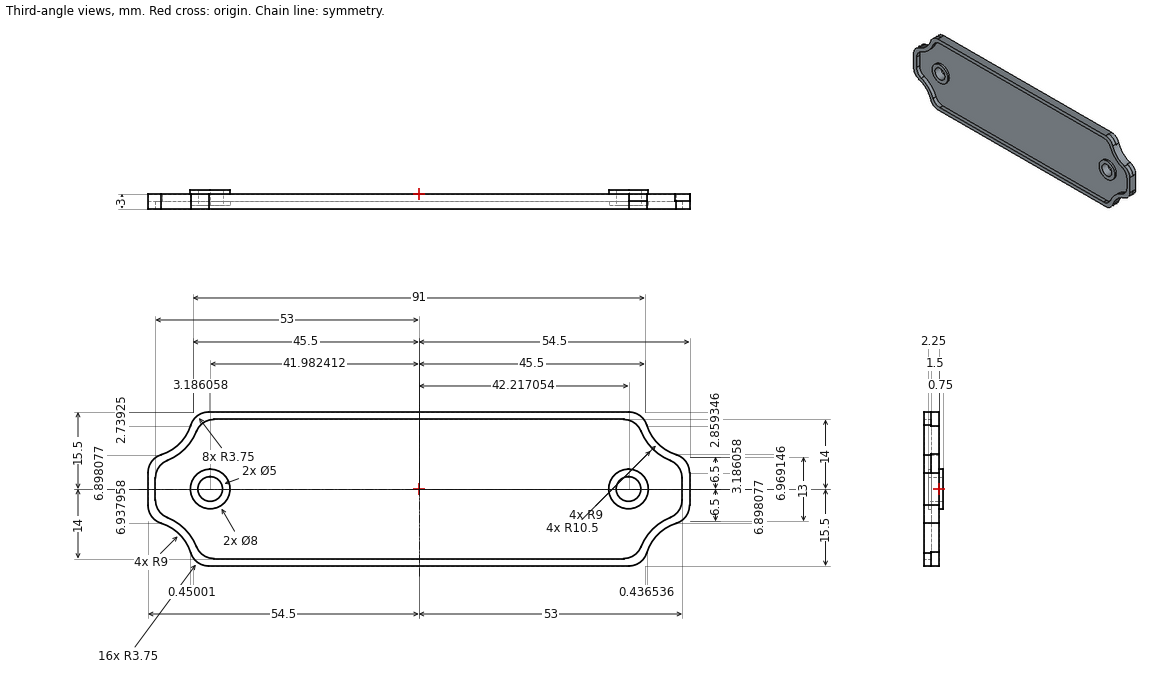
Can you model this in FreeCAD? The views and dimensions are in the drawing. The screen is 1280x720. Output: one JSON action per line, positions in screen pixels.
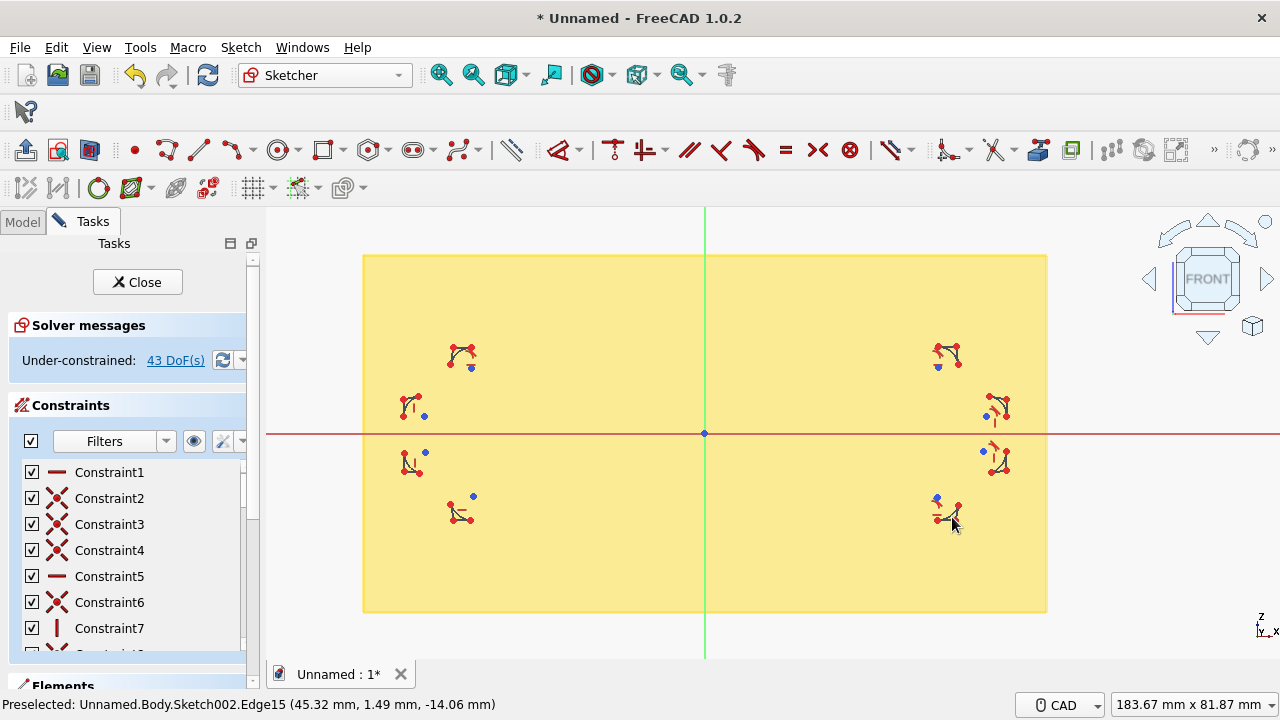
{"action": "scroll", "coordinate": [459, 520], "scroll_direction": "up", "scroll_amount": 7}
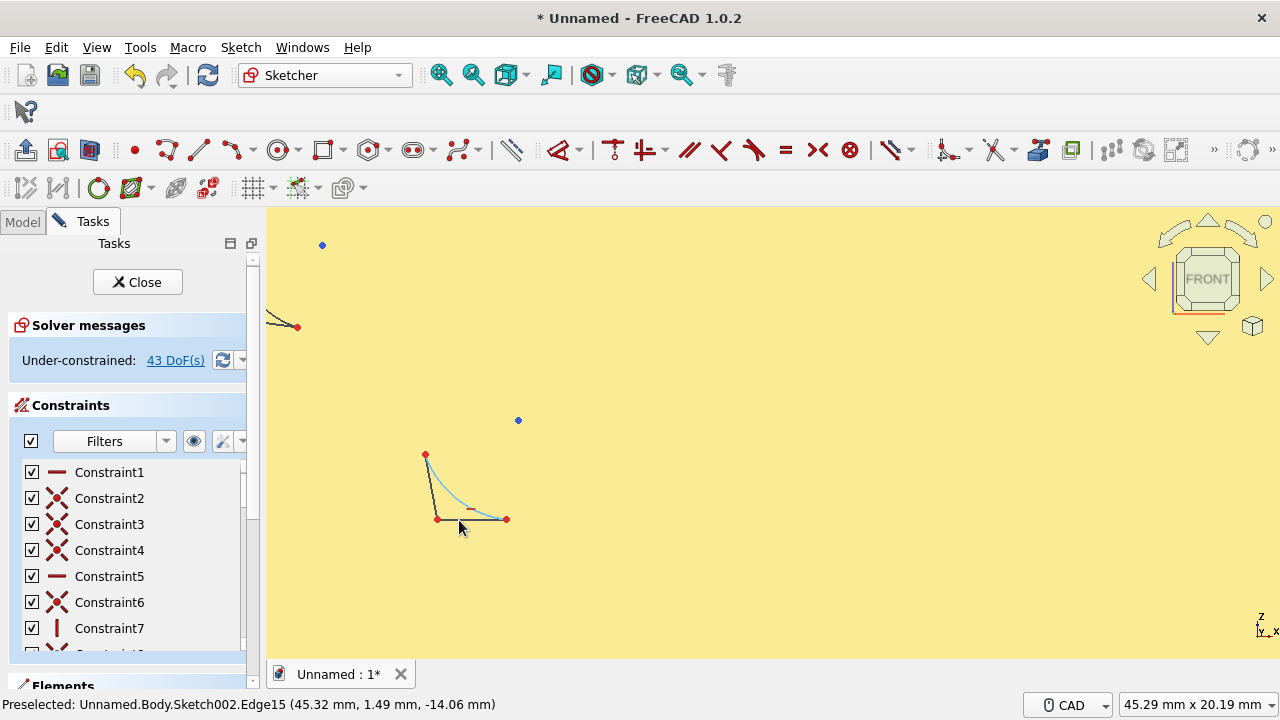
{"action": "left_click", "coordinate": [458, 520]}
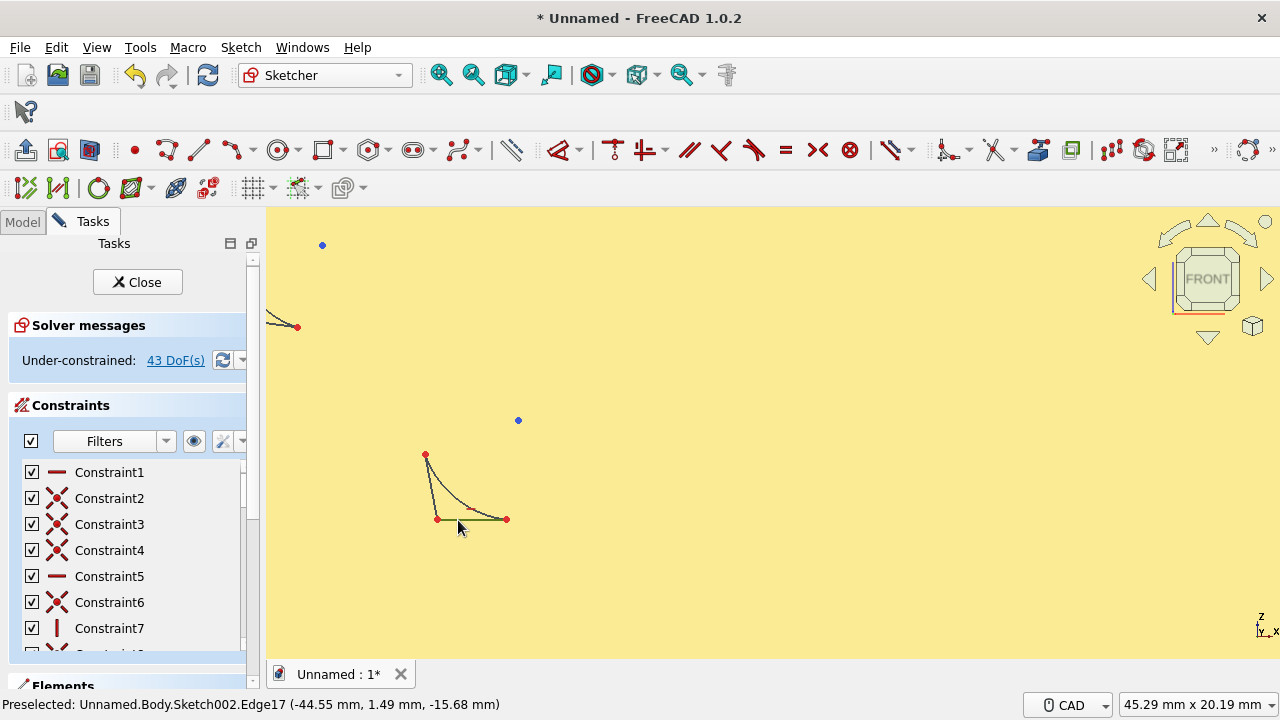
{"action": "scroll", "coordinate": [441, 483], "scroll_direction": "up", "scroll_amount": 2}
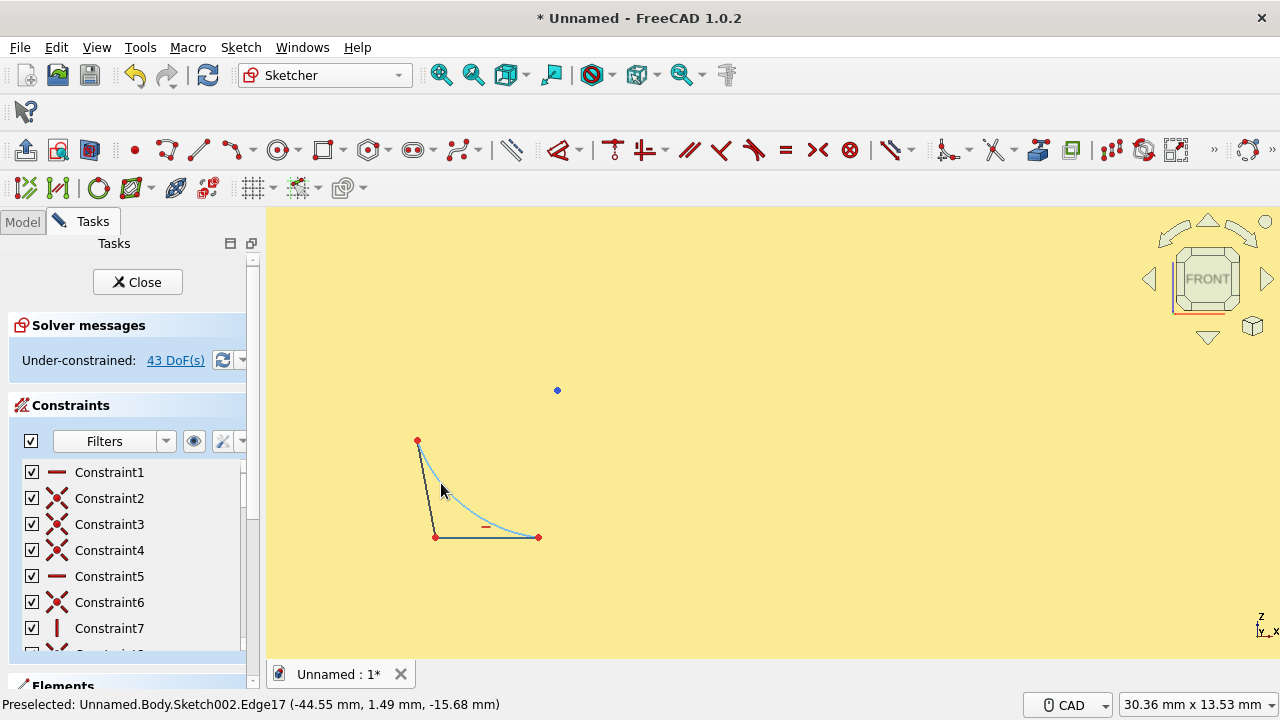
{"action": "left_click", "coordinate": [441, 483]}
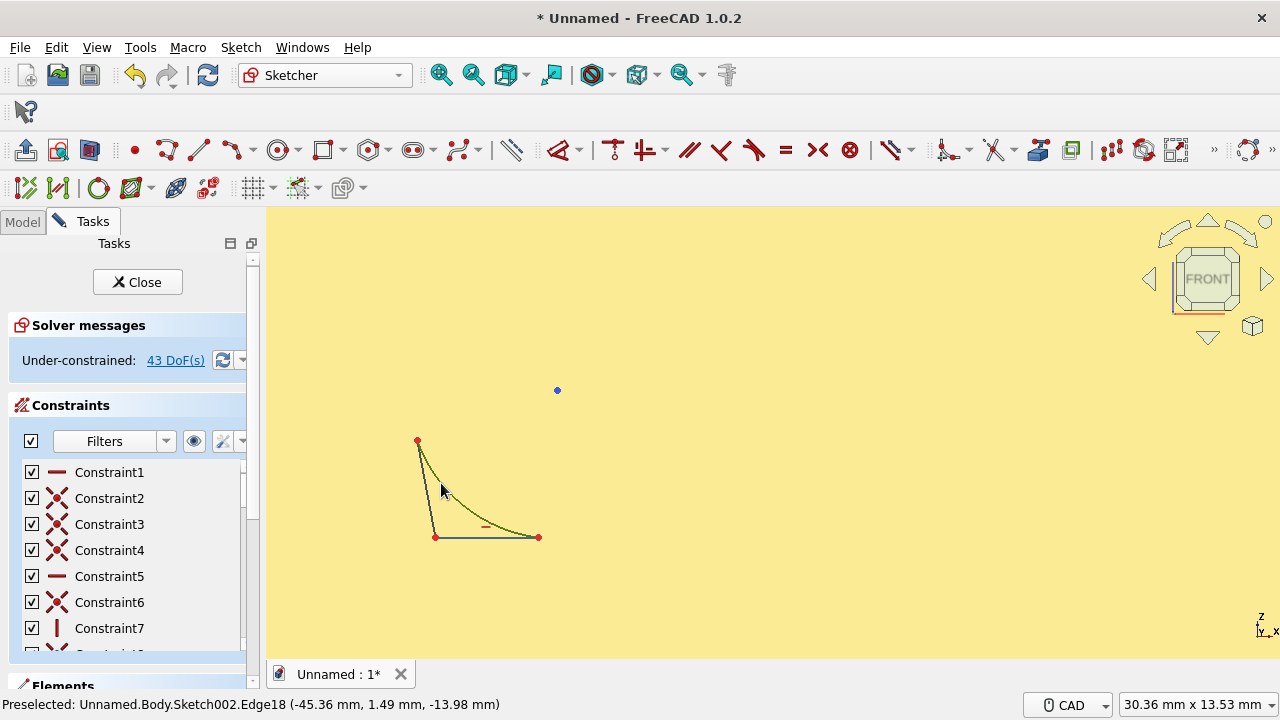
{"action": "left_click", "coordinate": [754, 150]}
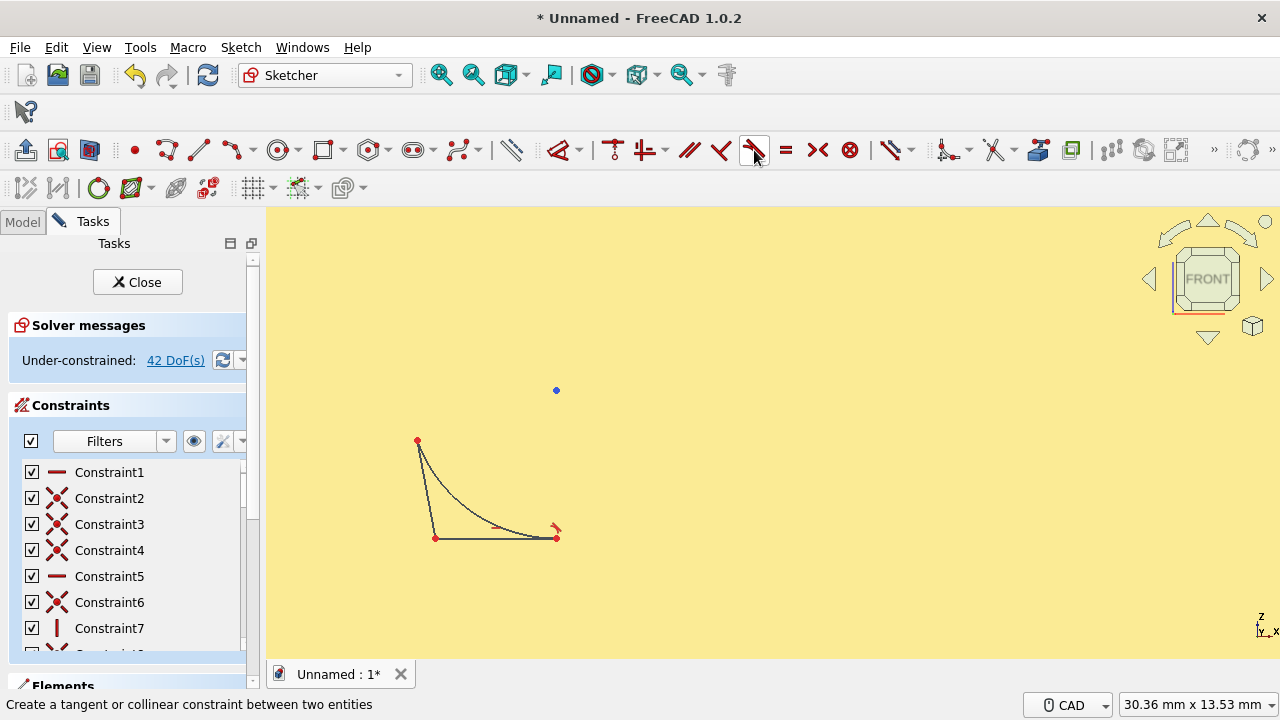
{"action": "scroll", "coordinate": [457, 516], "scroll_direction": "down", "scroll_amount": 9}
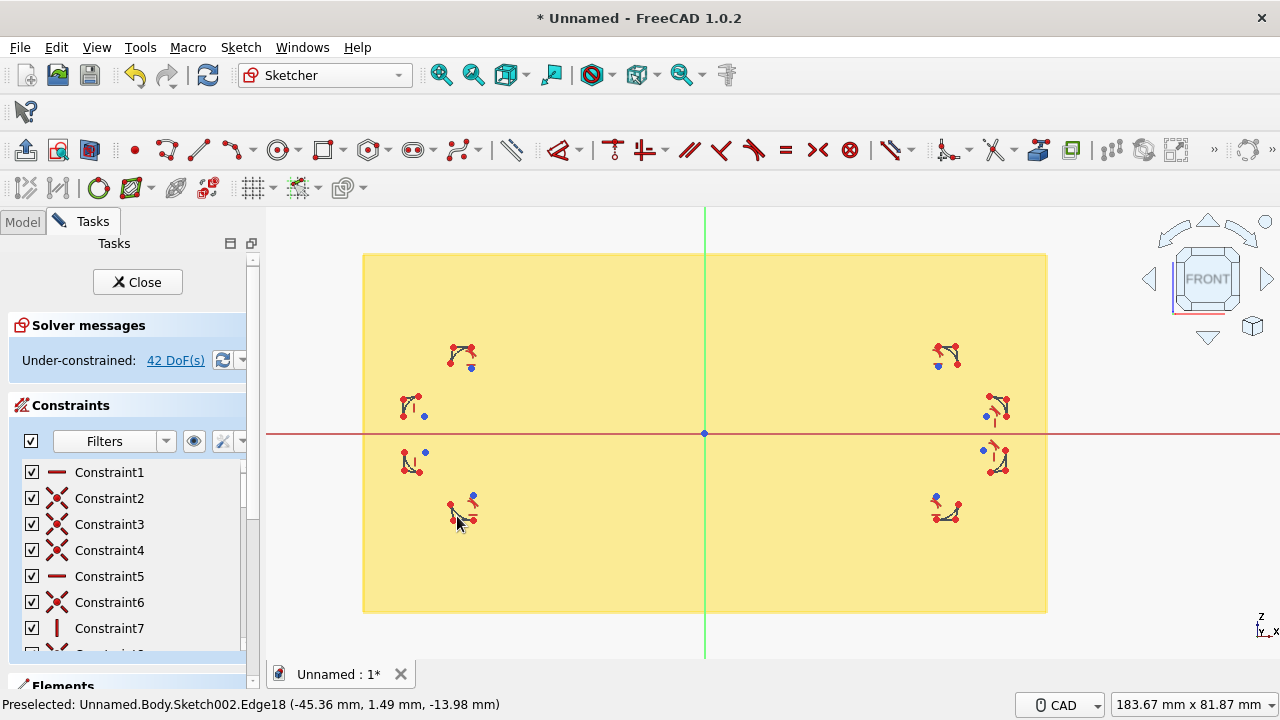
{"action": "scroll", "coordinate": [404, 465], "scroll_direction": "up", "scroll_amount": 7}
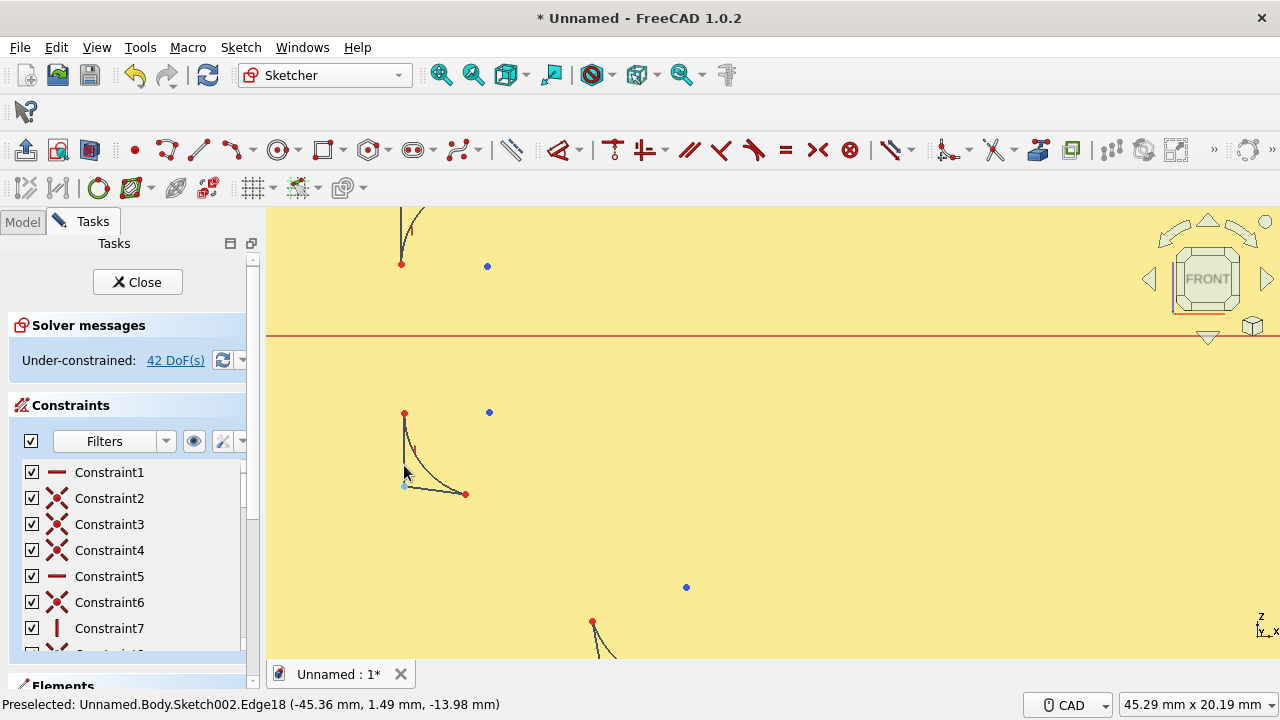
{"action": "left_click", "coordinate": [404, 464]}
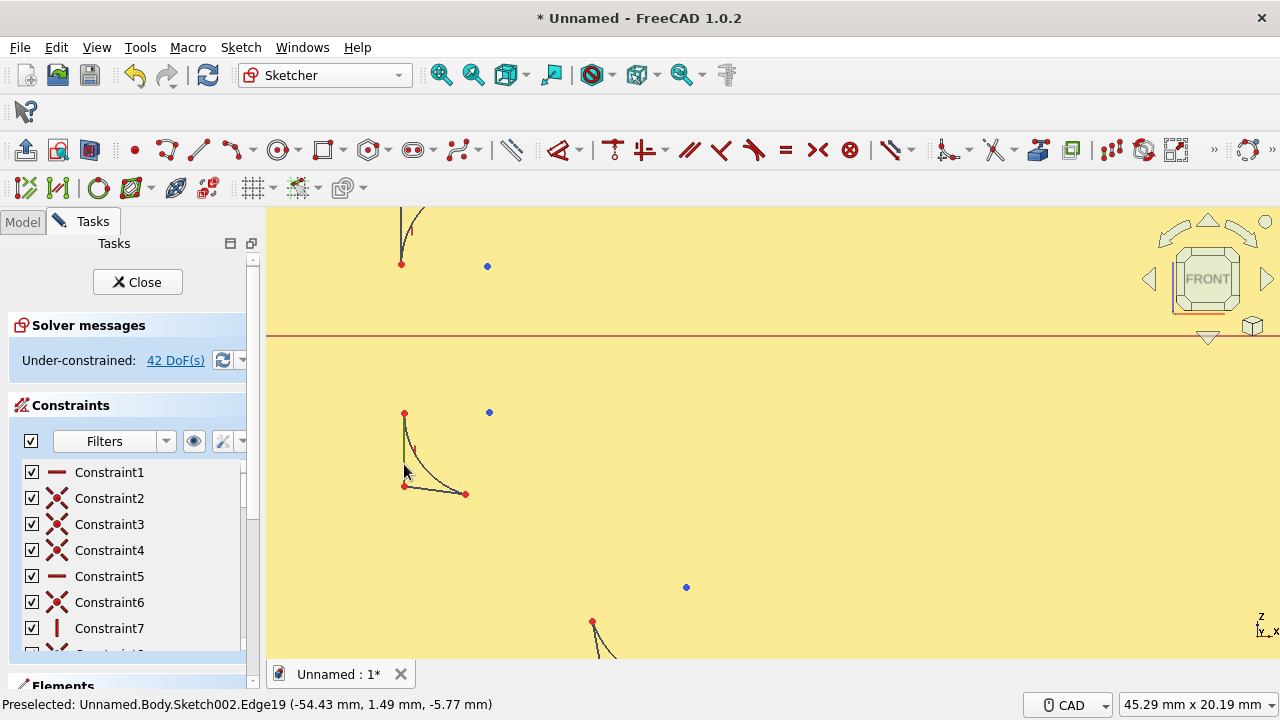
{"action": "scroll", "coordinate": [436, 479], "scroll_direction": "up", "scroll_amount": 2}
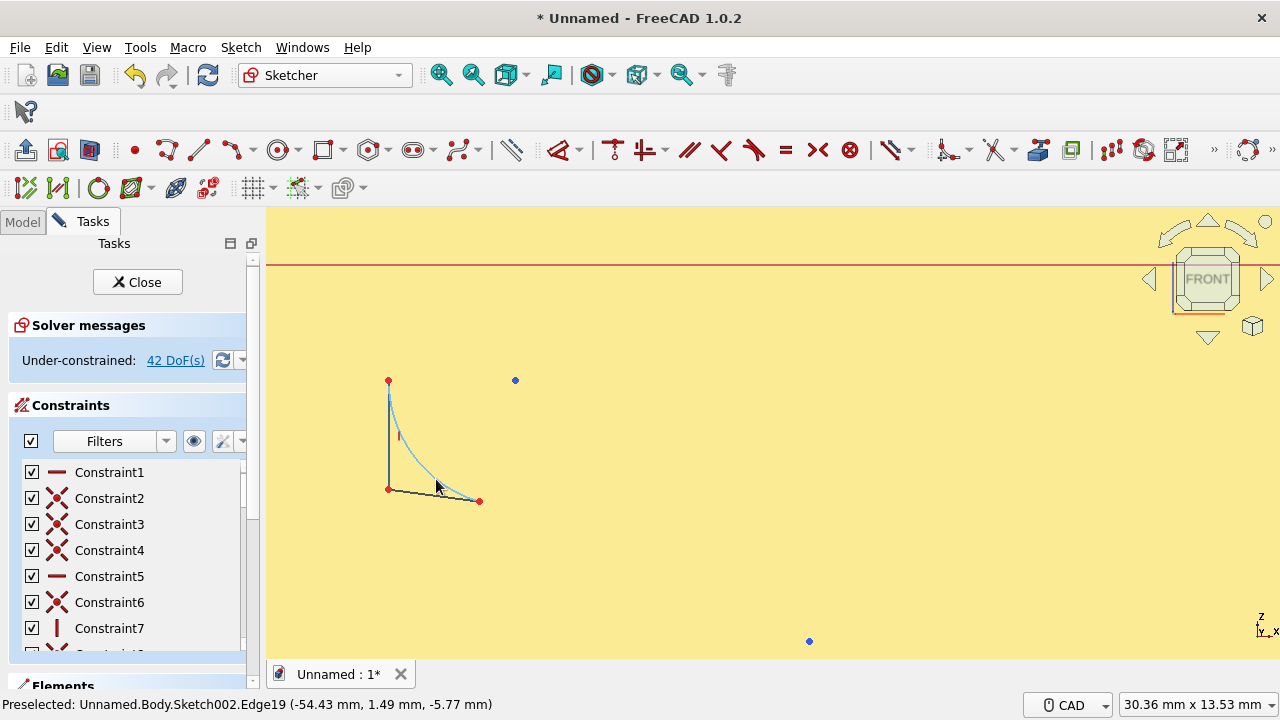
{"action": "left_click", "coordinate": [437, 479]}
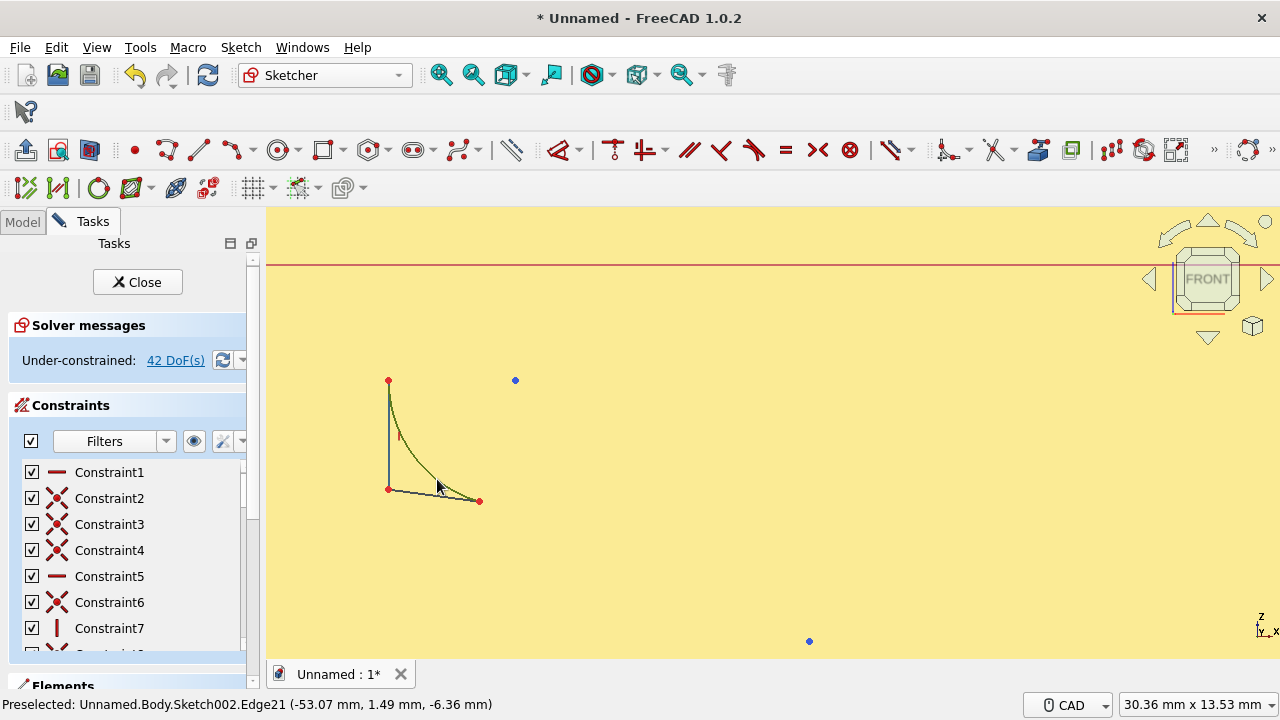
{"action": "left_click", "coordinate": [754, 150]}